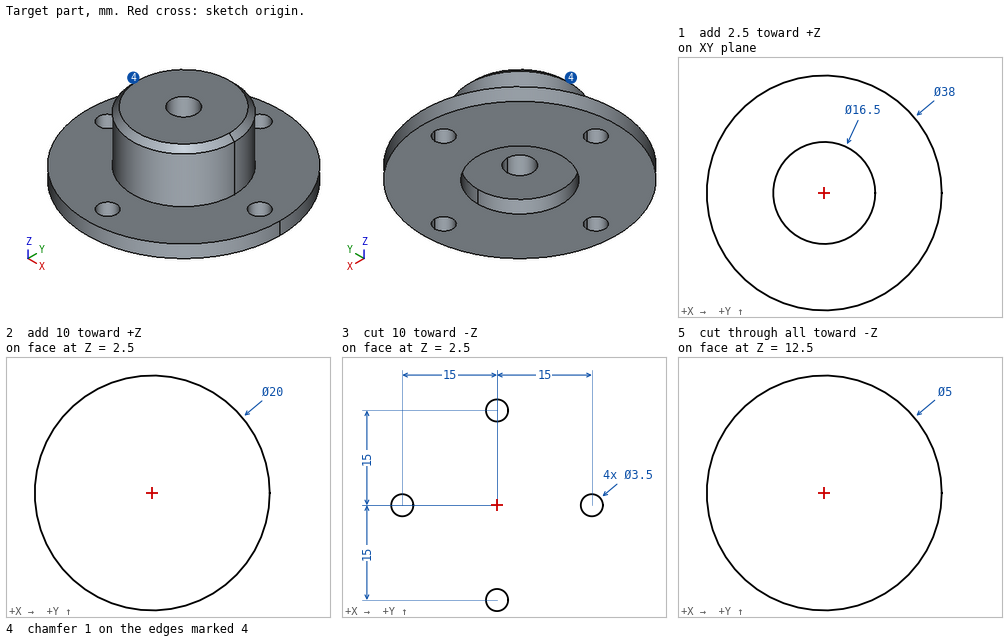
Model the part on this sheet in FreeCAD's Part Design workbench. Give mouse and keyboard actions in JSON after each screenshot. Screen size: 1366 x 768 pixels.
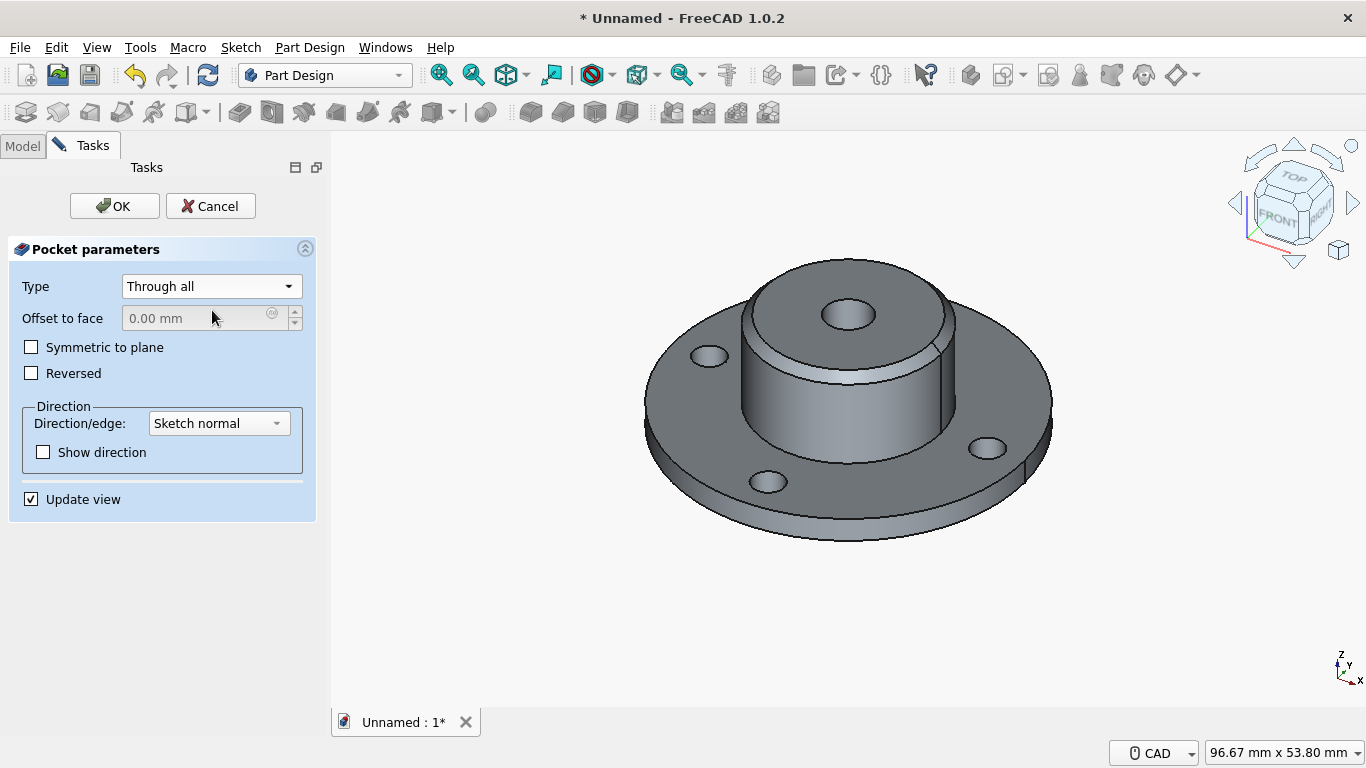
{"action": "left_click", "coordinate": [115, 206]}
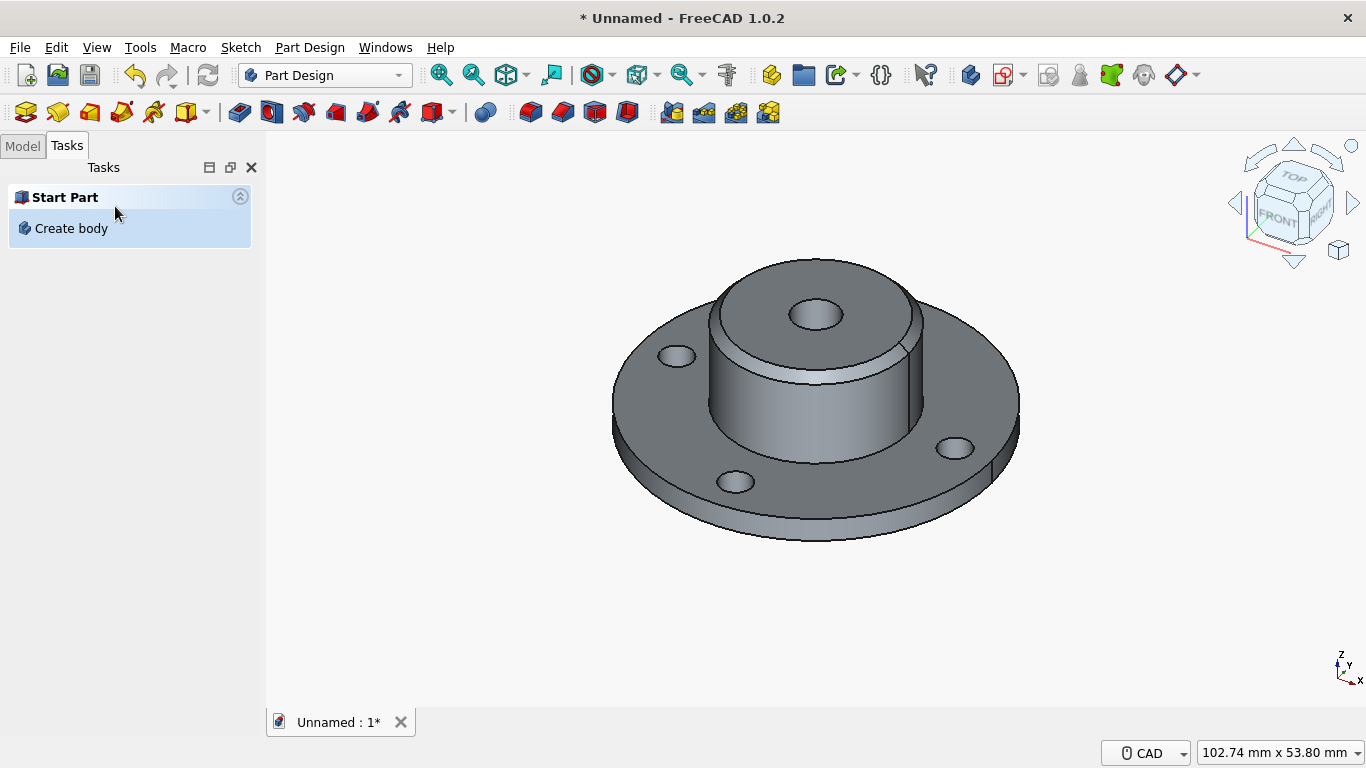
{"action": "key", "text": "0"}